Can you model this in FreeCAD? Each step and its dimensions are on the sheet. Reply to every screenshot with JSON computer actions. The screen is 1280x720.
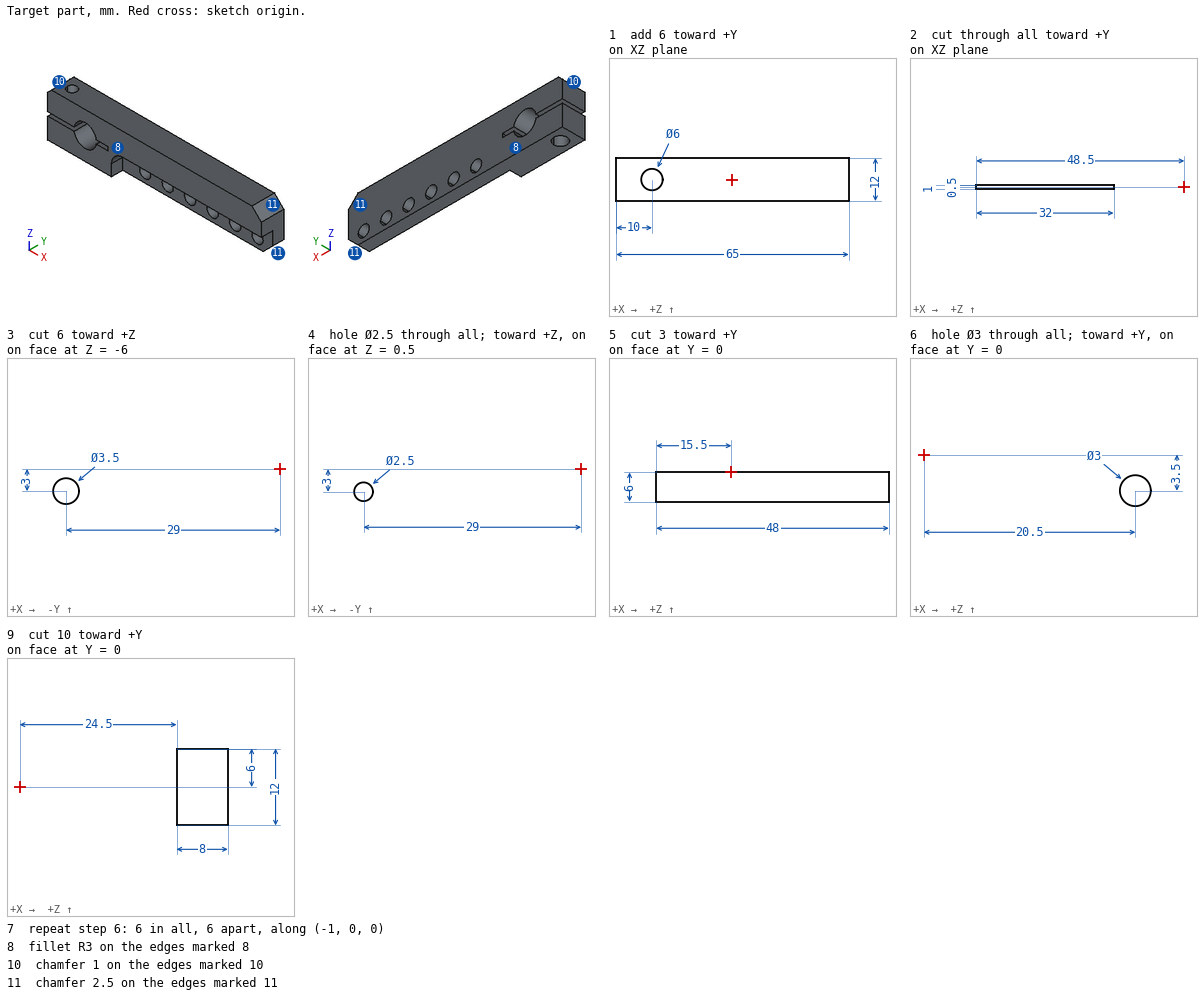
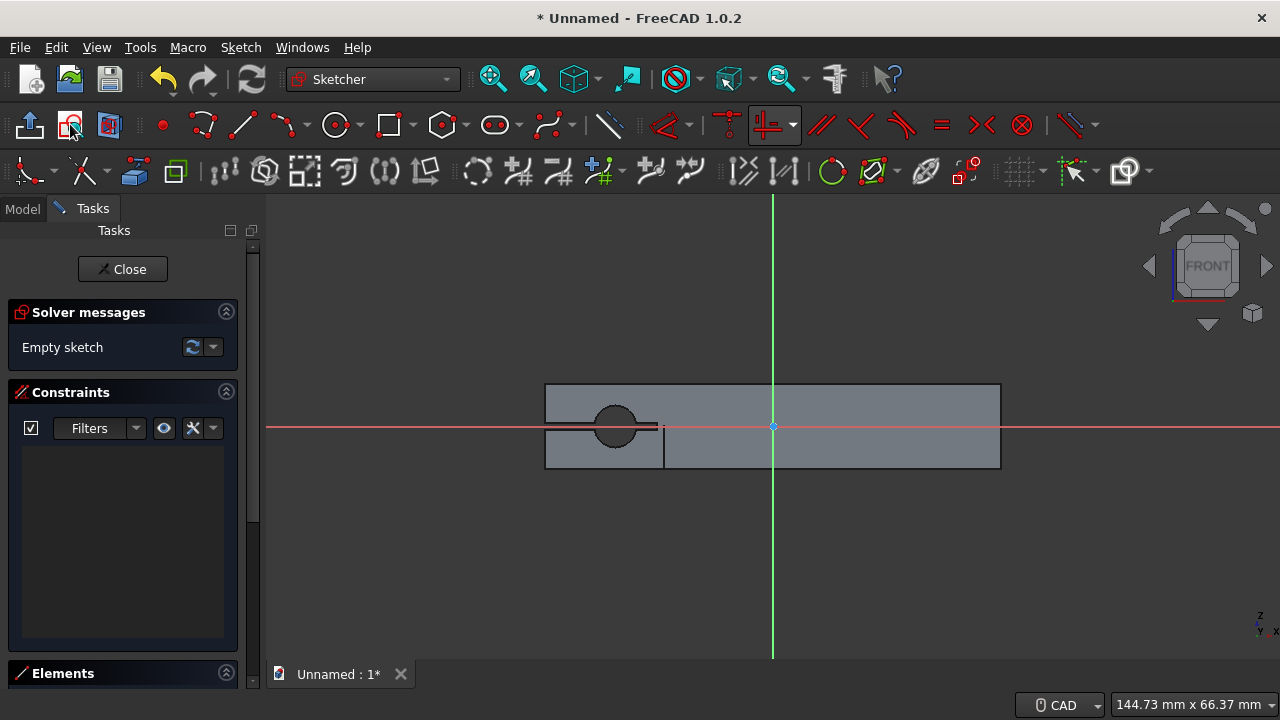
{"action": "scroll", "coordinate": [934, 453], "scroll_direction": "up", "scroll_amount": 13}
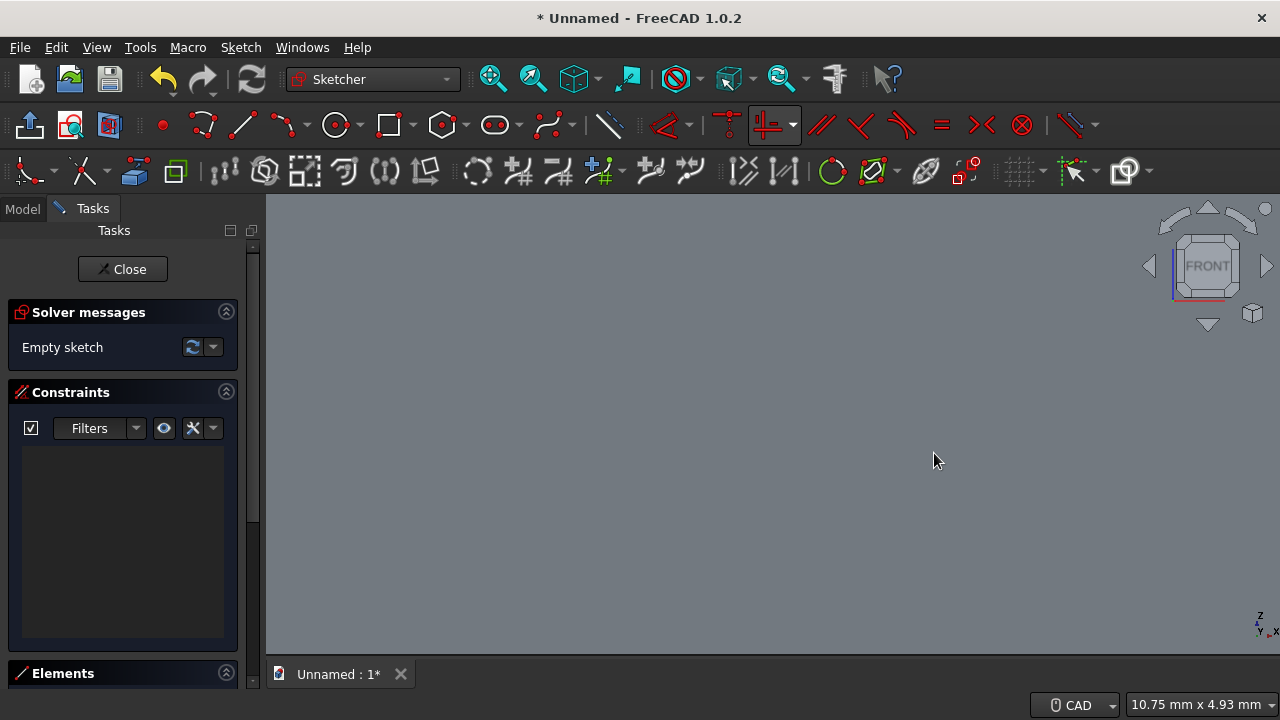
{"action": "left_click", "coordinate": [336, 126]}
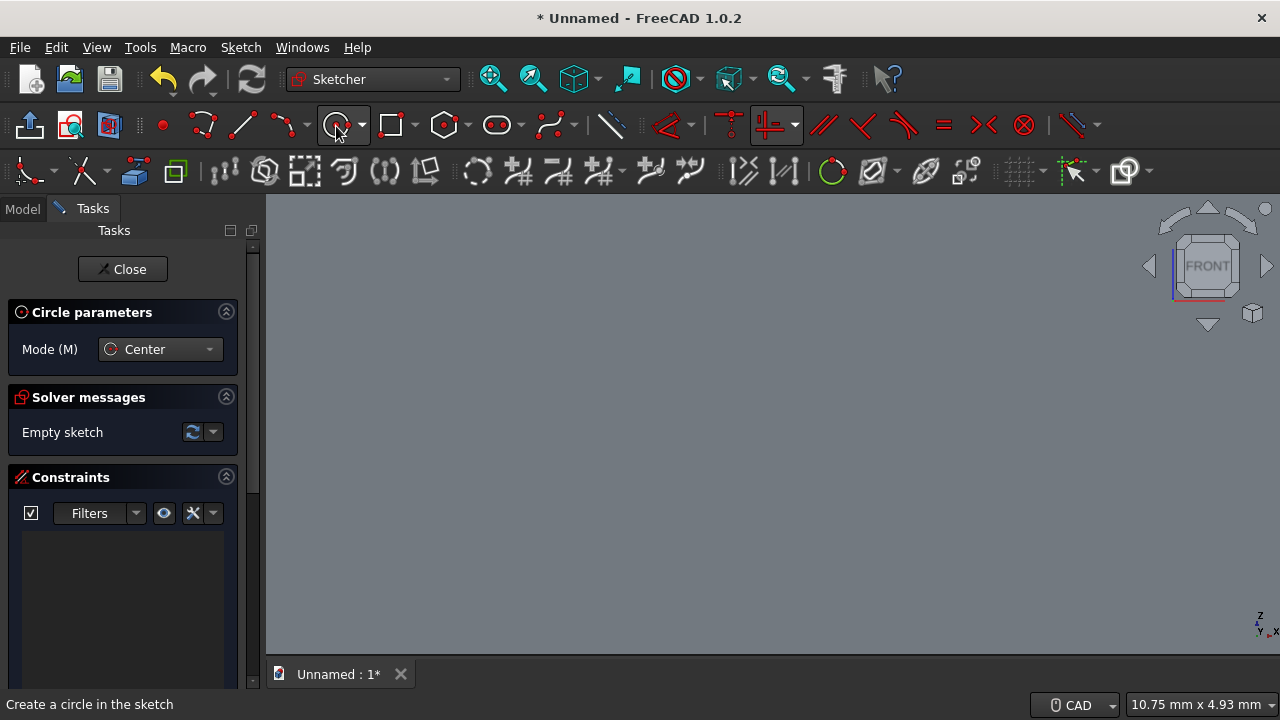
{"action": "left_click", "coordinate": [692, 419]}
{"action": "left_click", "coordinate": [792, 319]}
{"action": "key", "text": "Escape"}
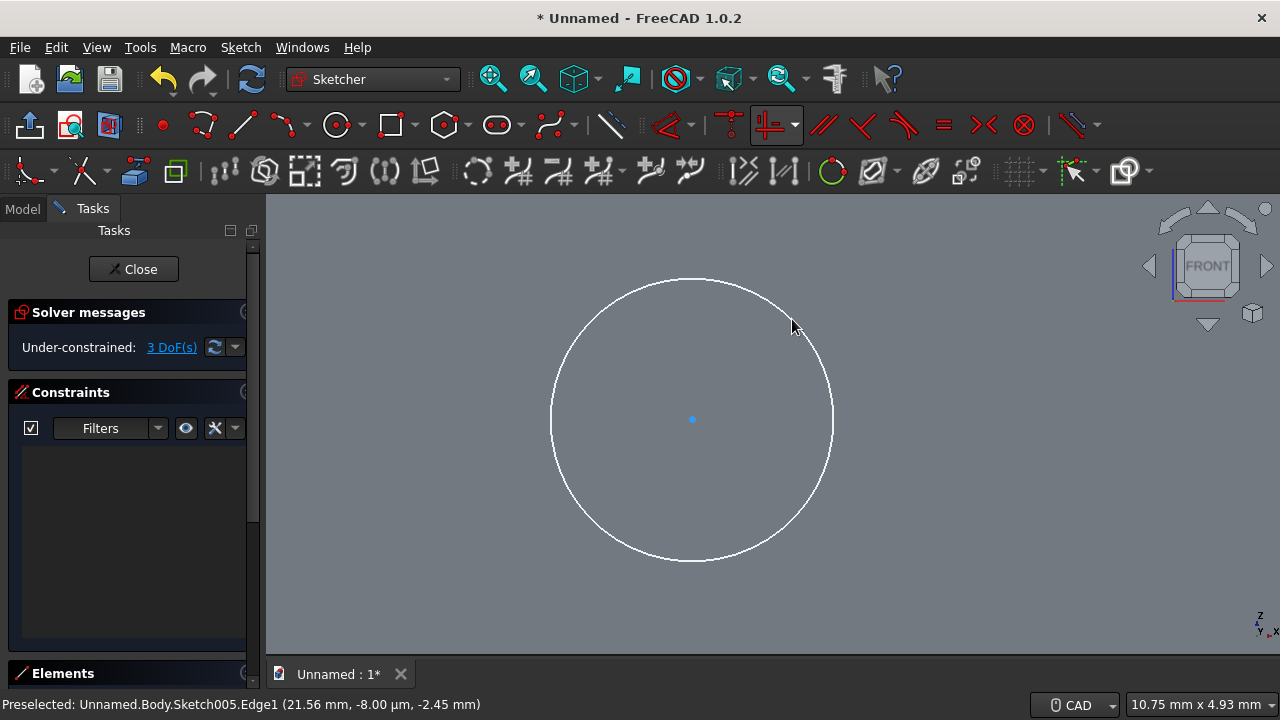
{"action": "left_click", "coordinate": [666, 126]}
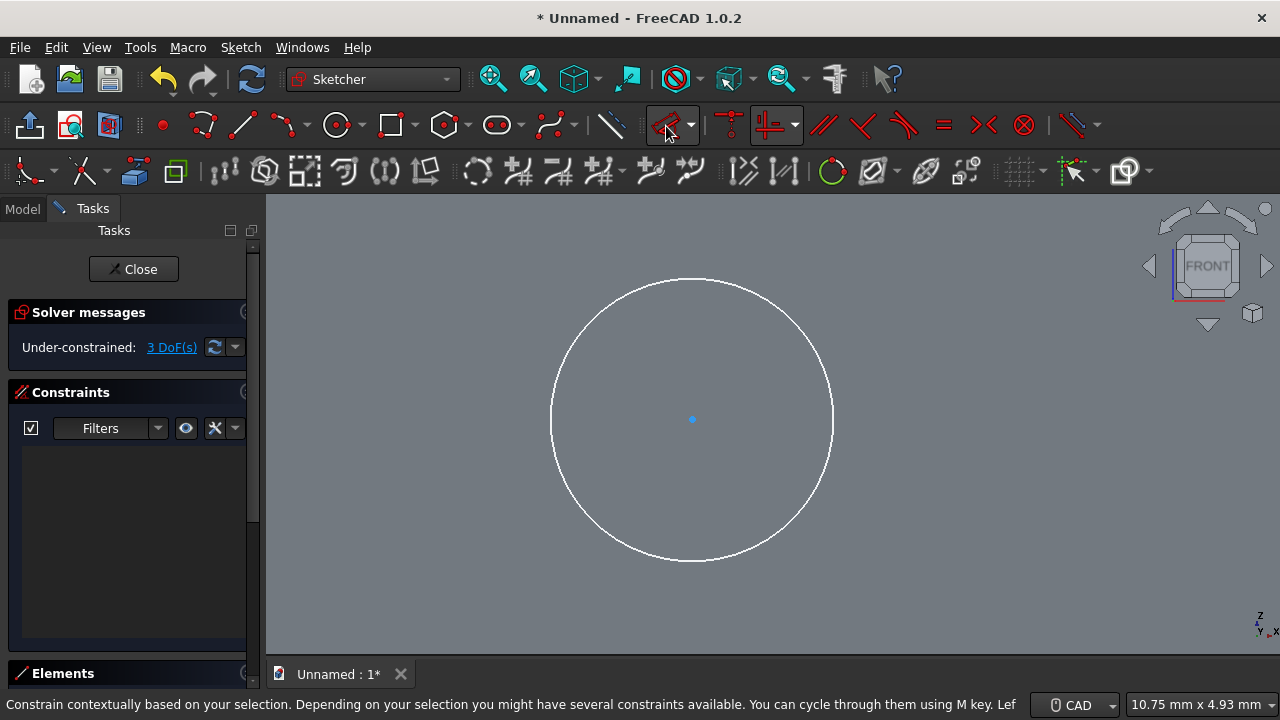
{"action": "left_click", "coordinate": [792, 320]}
{"action": "left_click", "coordinate": [815, 297]}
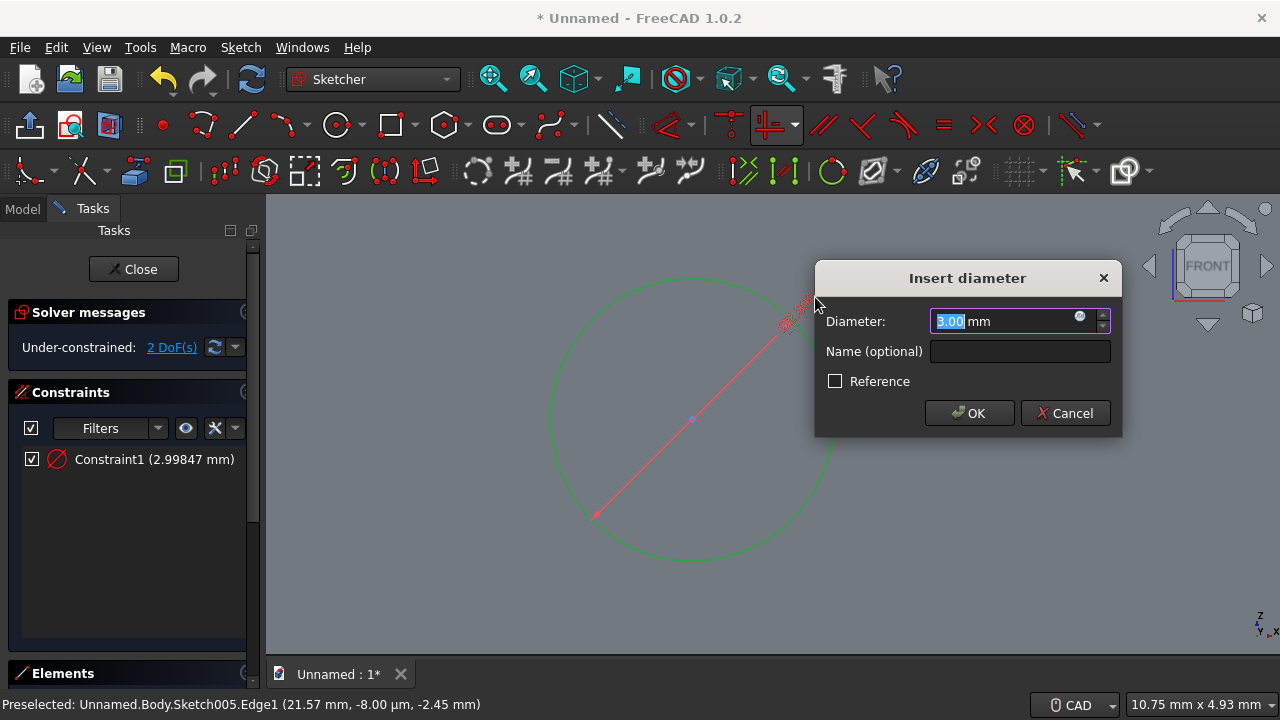
{"action": "type", "text": "3"}
{"action": "key", "text": "Return"}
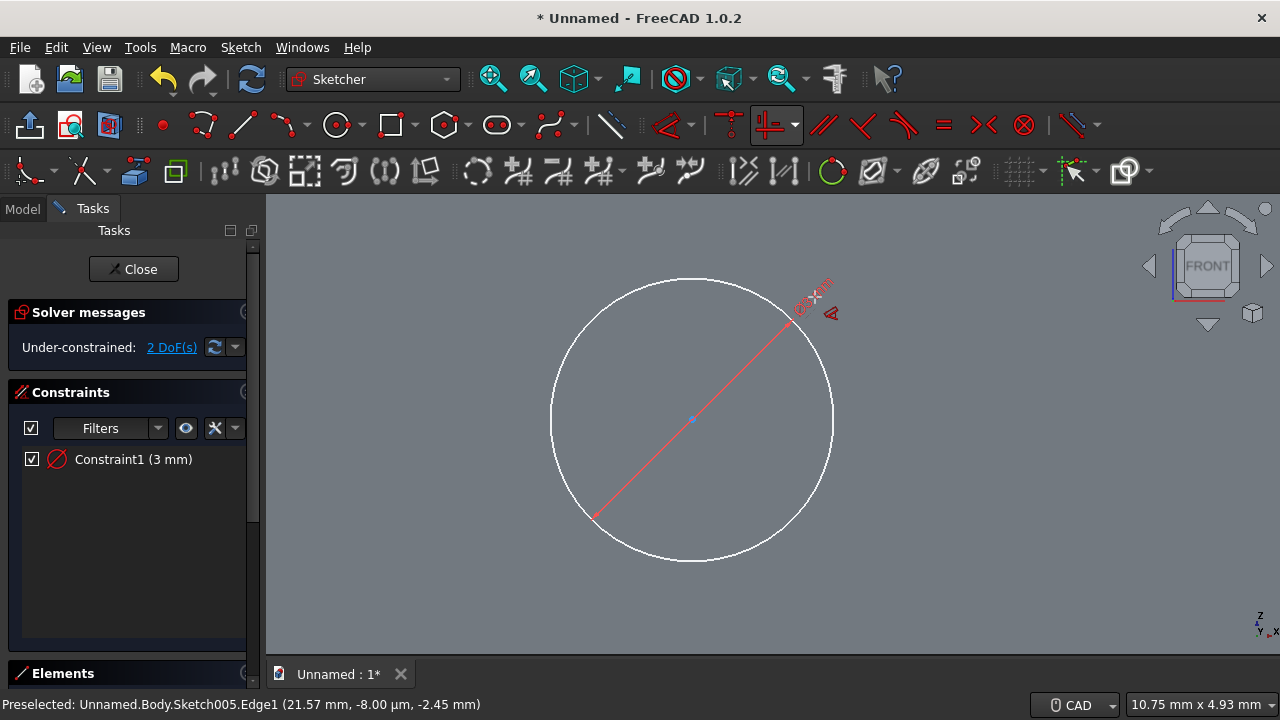
{"action": "left_click", "coordinate": [692, 420]}
{"action": "left_click", "coordinate": [726, 321]}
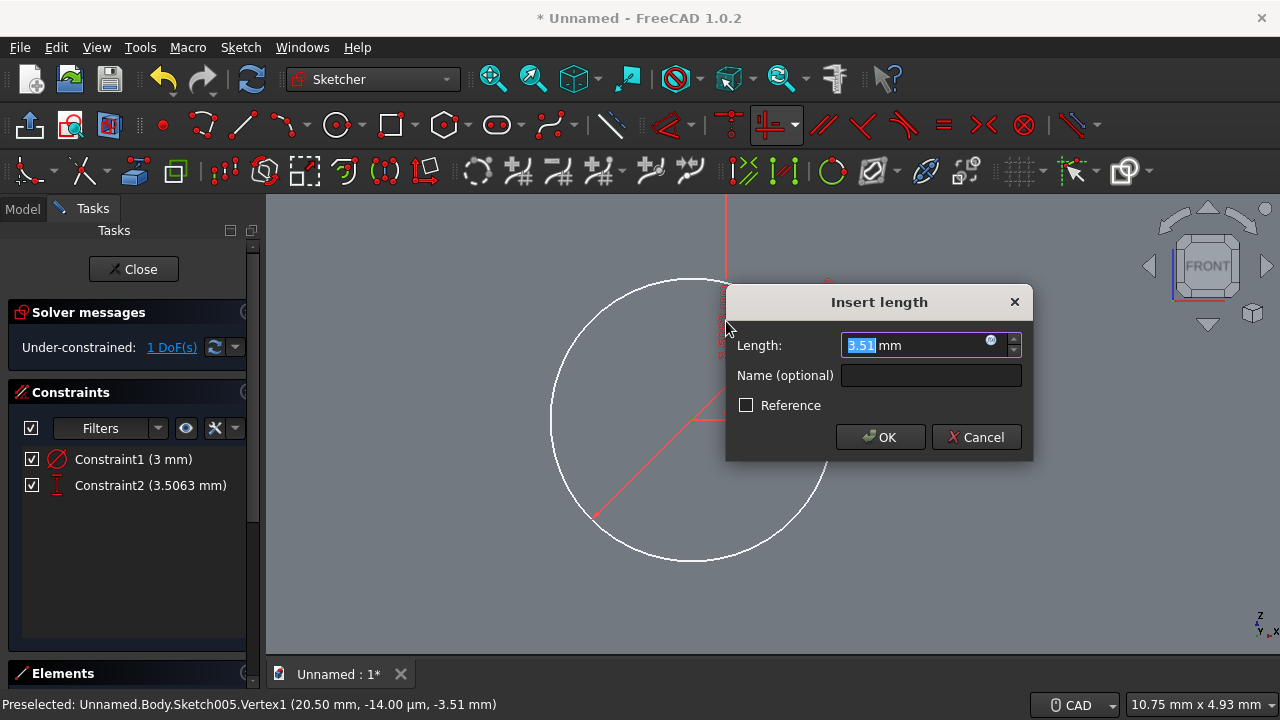
{"action": "type", "text": "3.5"}
{"action": "key", "text": "Return"}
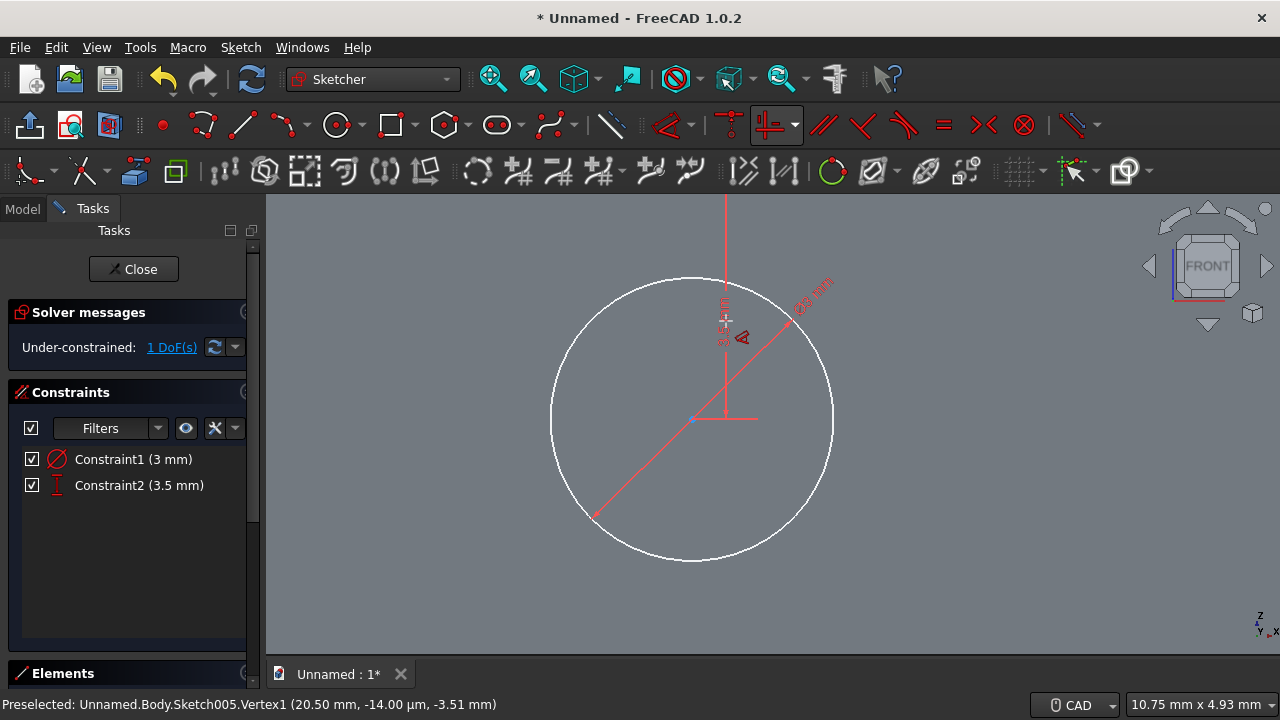
{"action": "left_click", "coordinate": [692, 419]}
{"action": "left_click", "coordinate": [493, 453]}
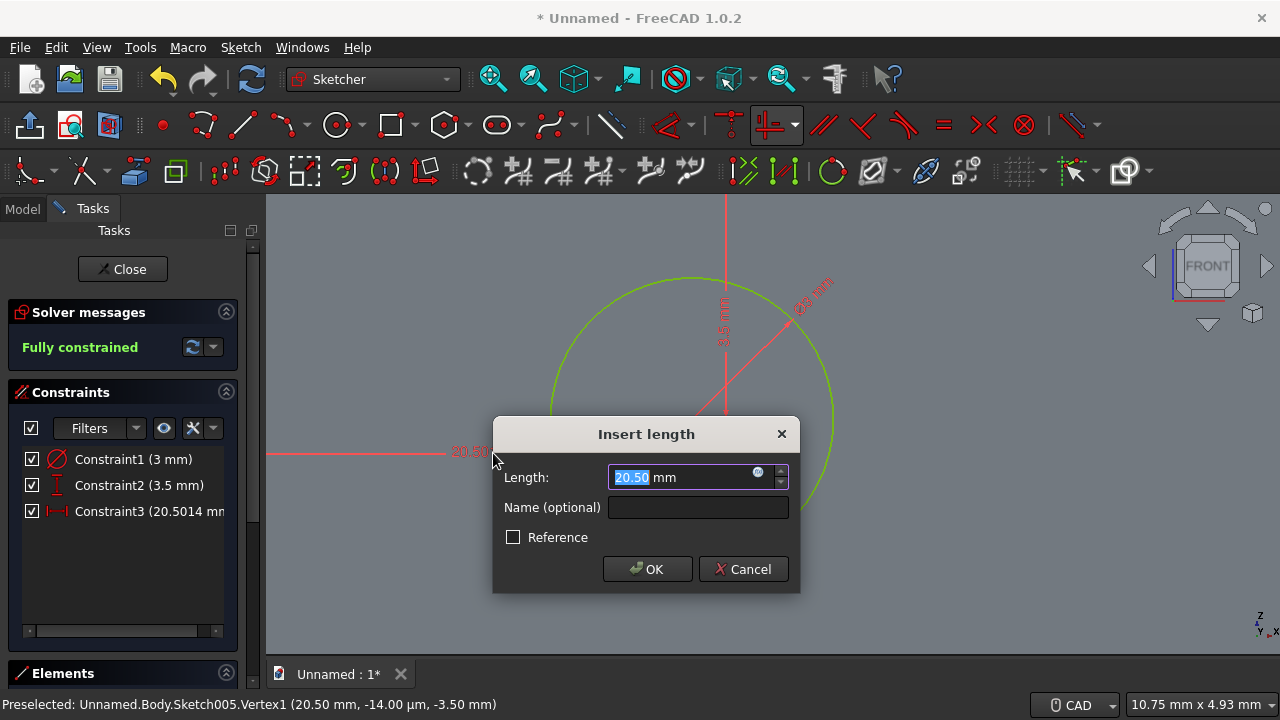
{"action": "type", "text": "20.5"}
{"action": "key", "text": "Return"}
{"action": "key", "text": "Escape"}